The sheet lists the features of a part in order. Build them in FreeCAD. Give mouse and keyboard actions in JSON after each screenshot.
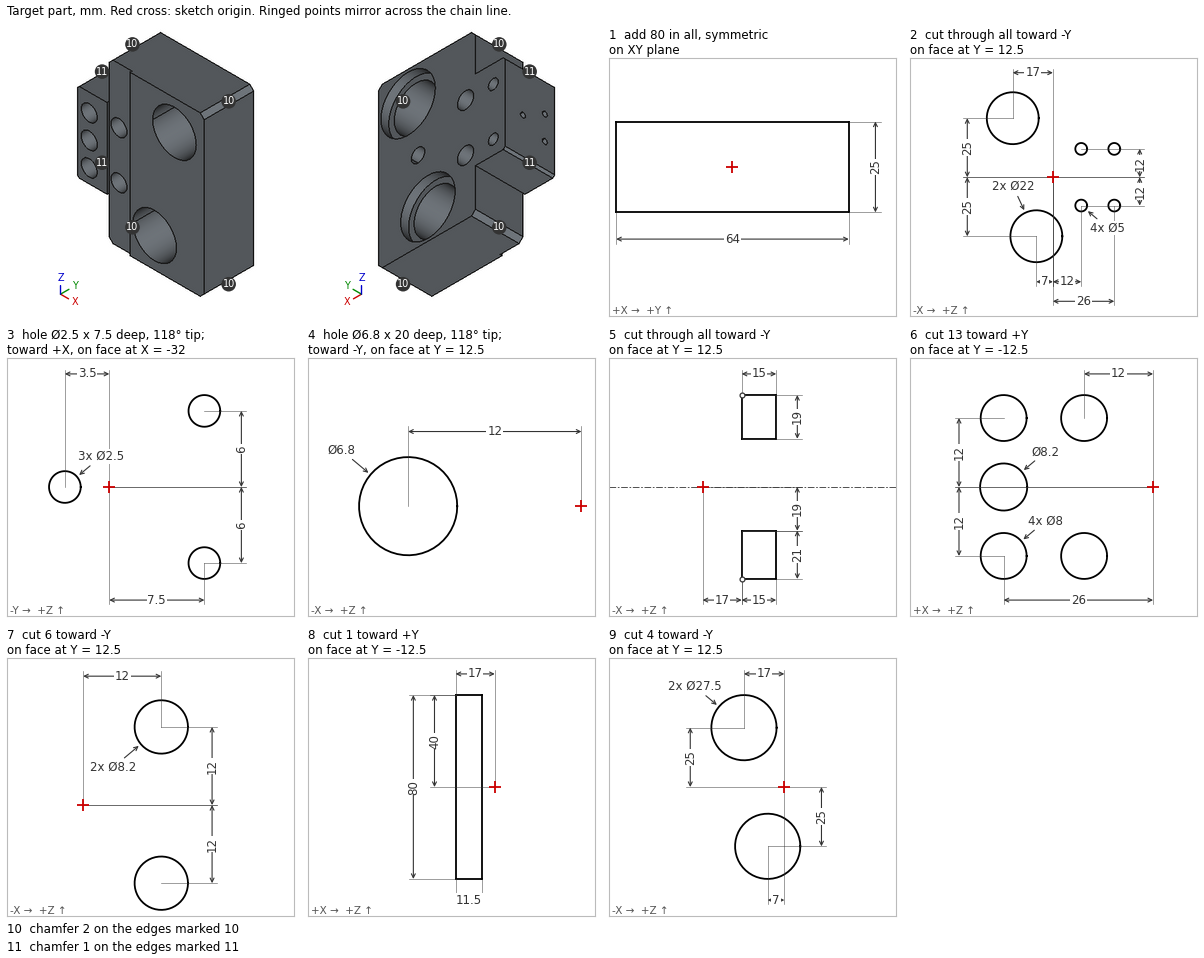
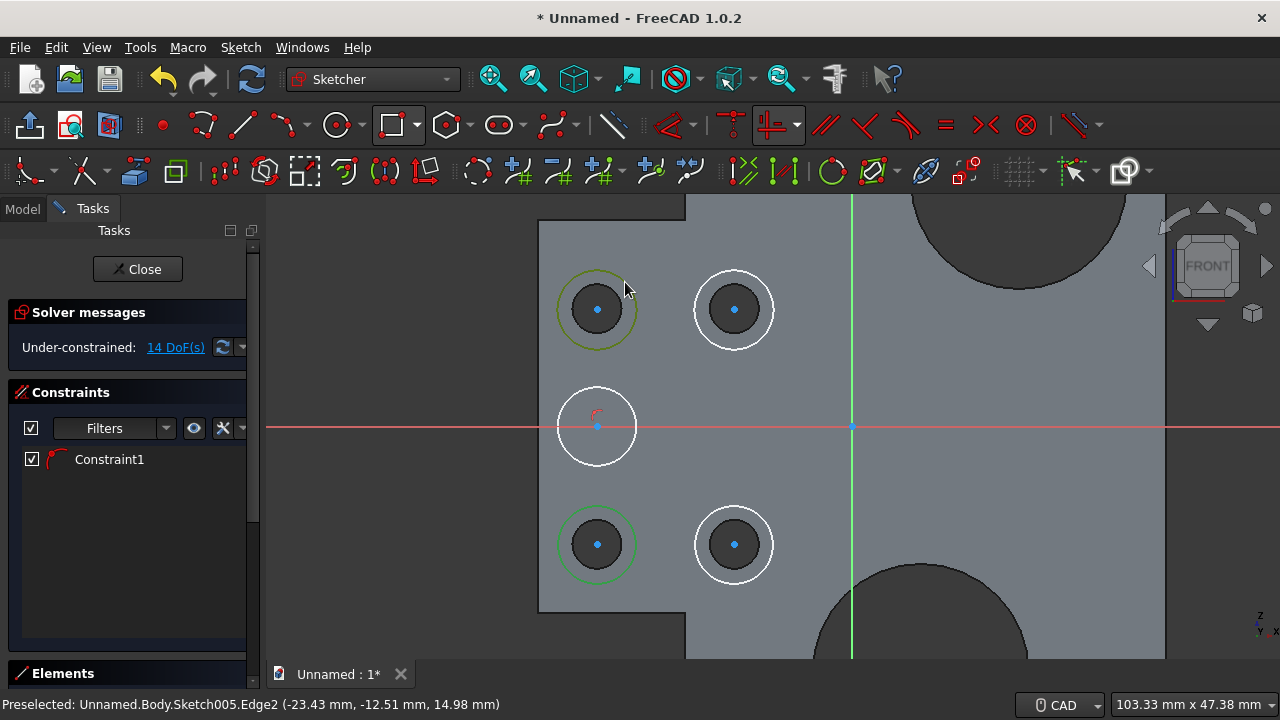
{"action": "left_click", "coordinate": [762, 282]}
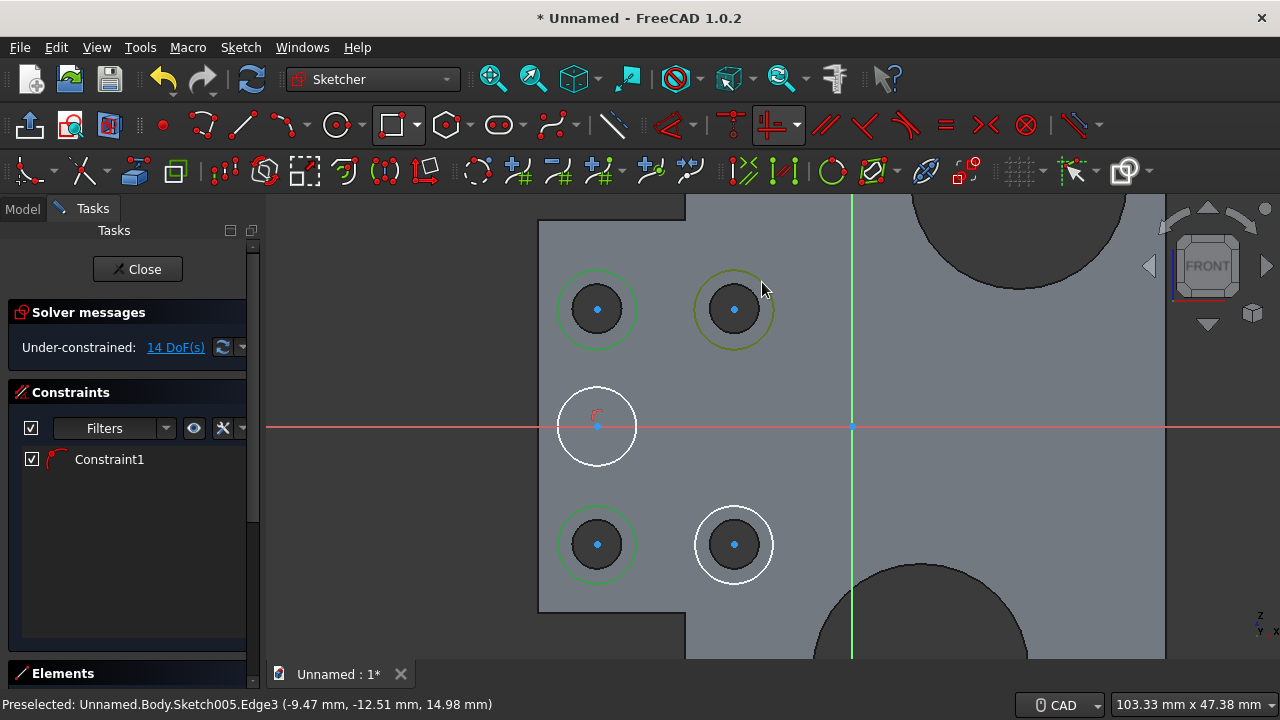
{"action": "left_click", "coordinate": [761, 517]}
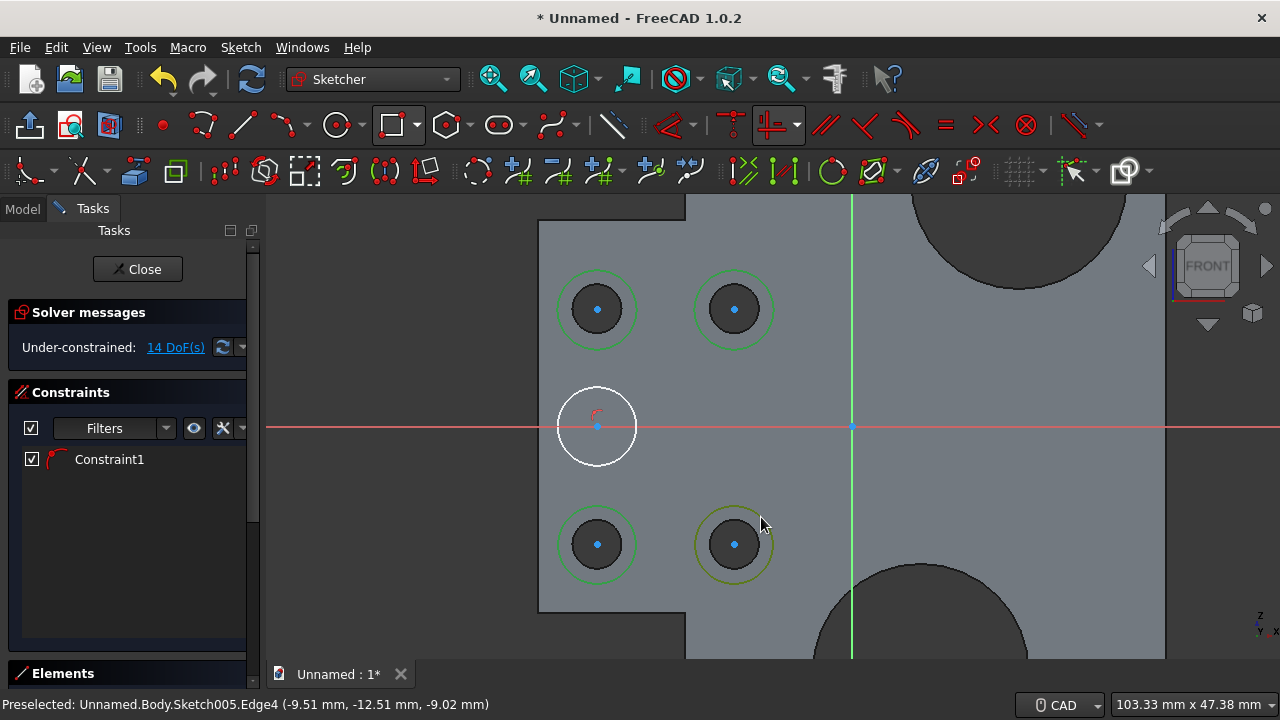
{"action": "left_click", "coordinate": [946, 126]}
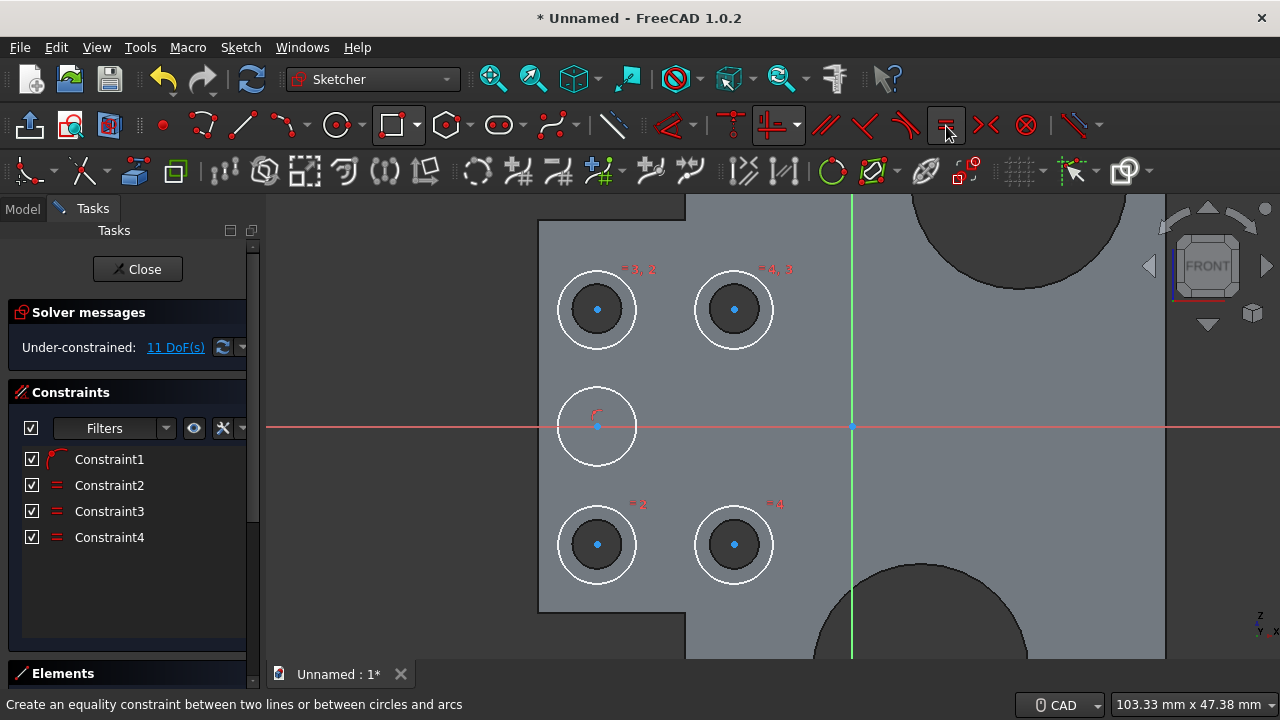
{"action": "left_click", "coordinate": [597, 545]}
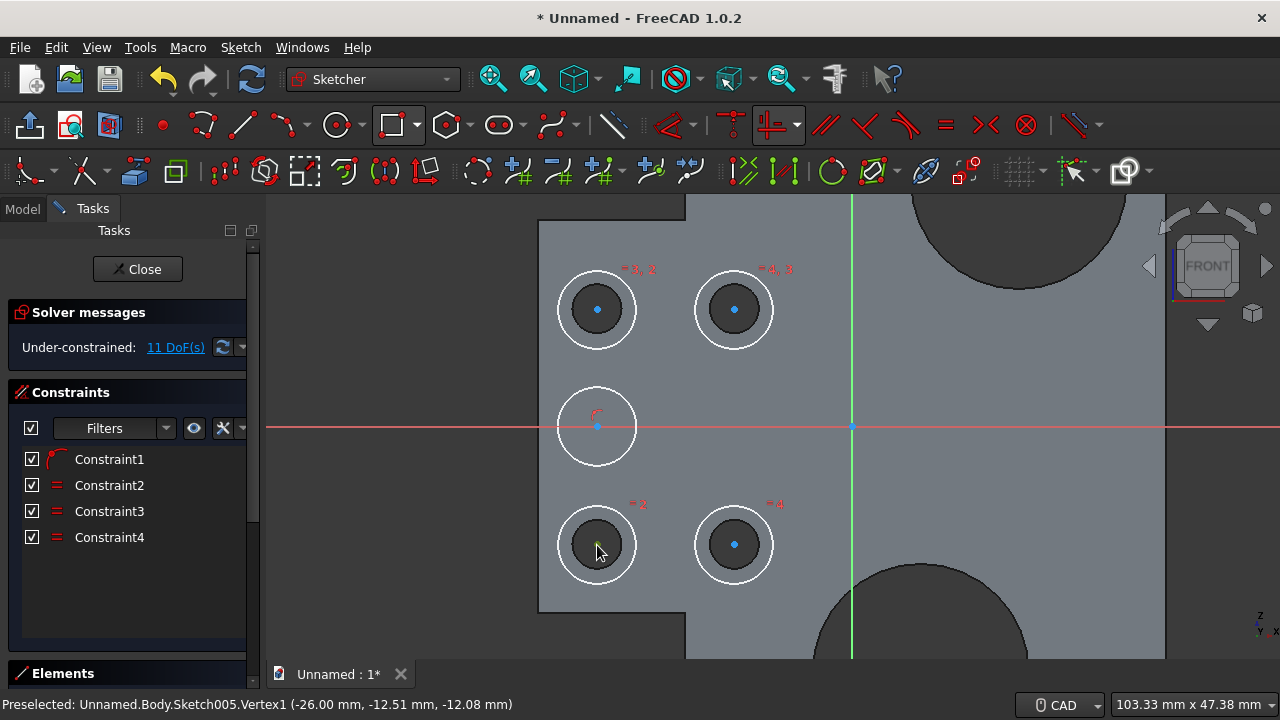
{"action": "left_click", "coordinate": [597, 310]}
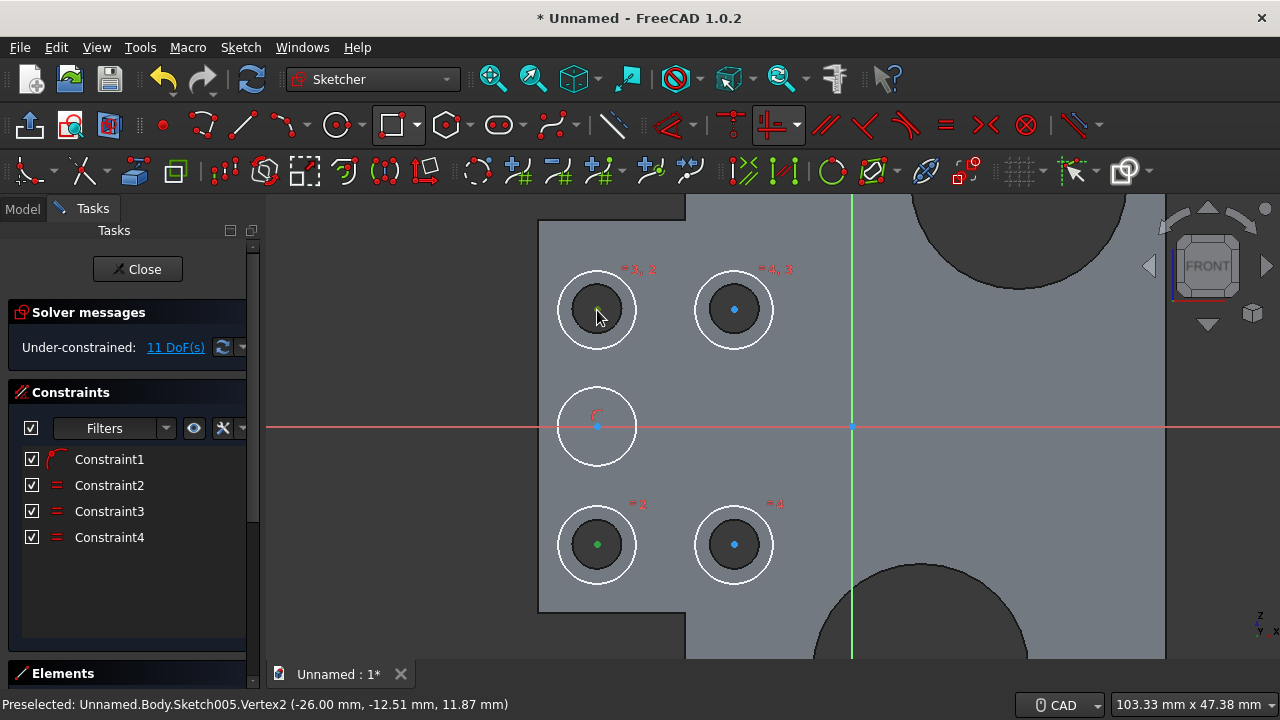
{"action": "left_click", "coordinate": [800, 126]}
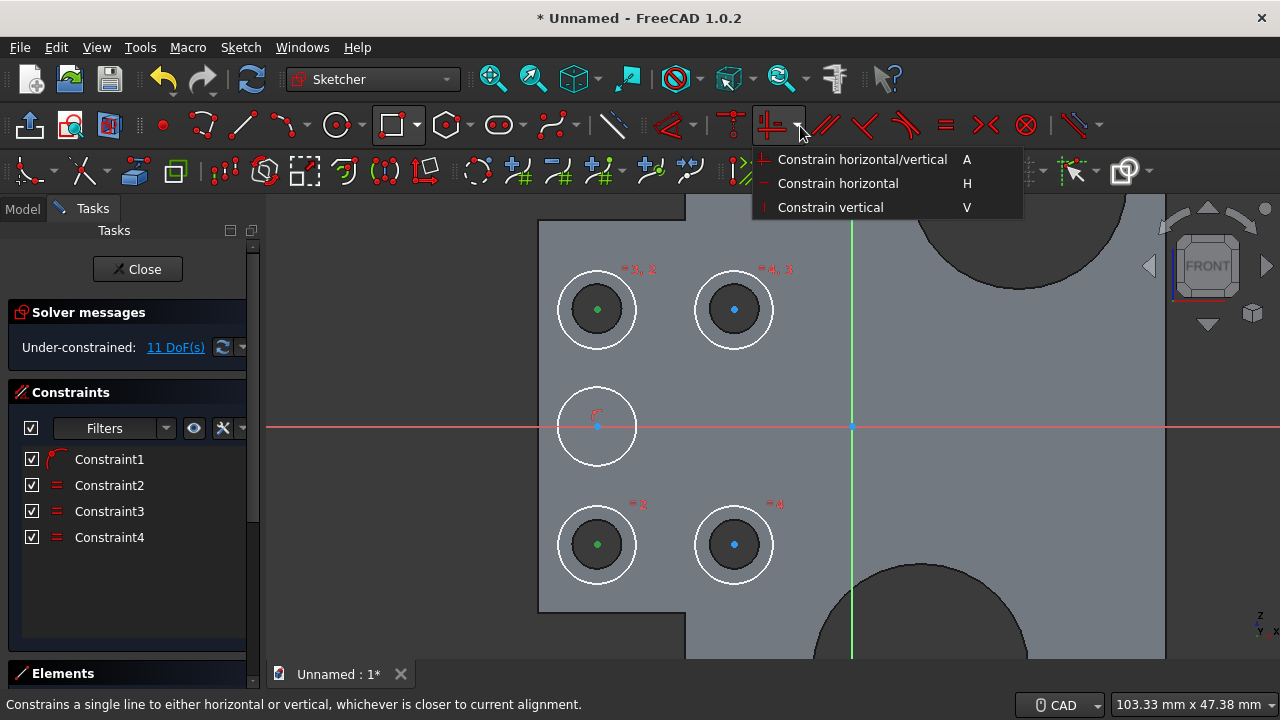
{"action": "left_click", "coordinate": [888, 207]}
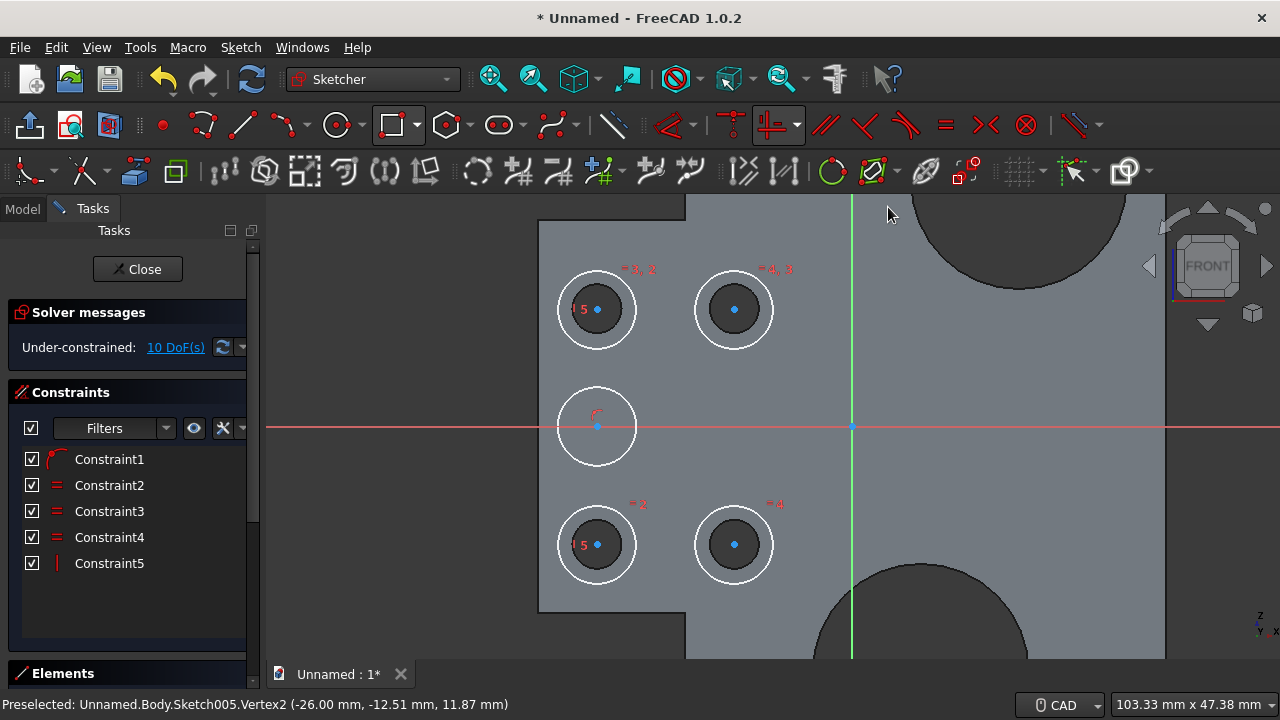
{"action": "left_click", "coordinate": [597, 310]}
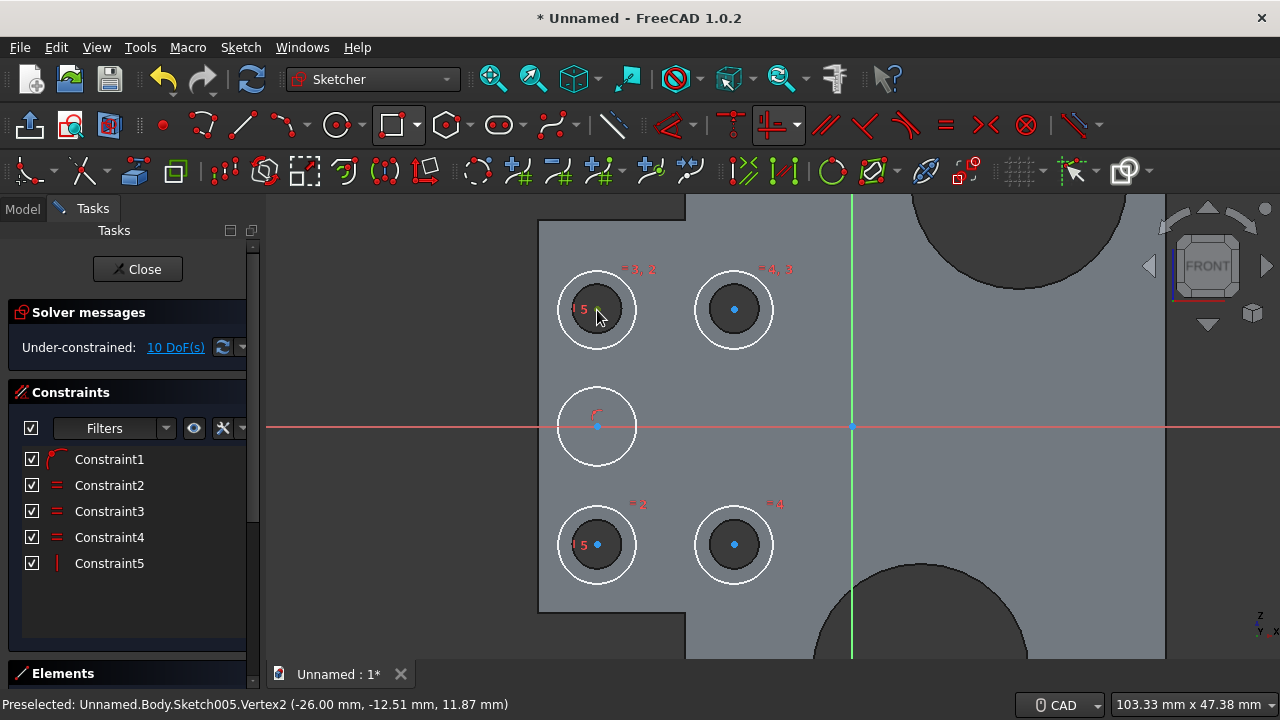
{"action": "left_click", "coordinate": [734, 310]}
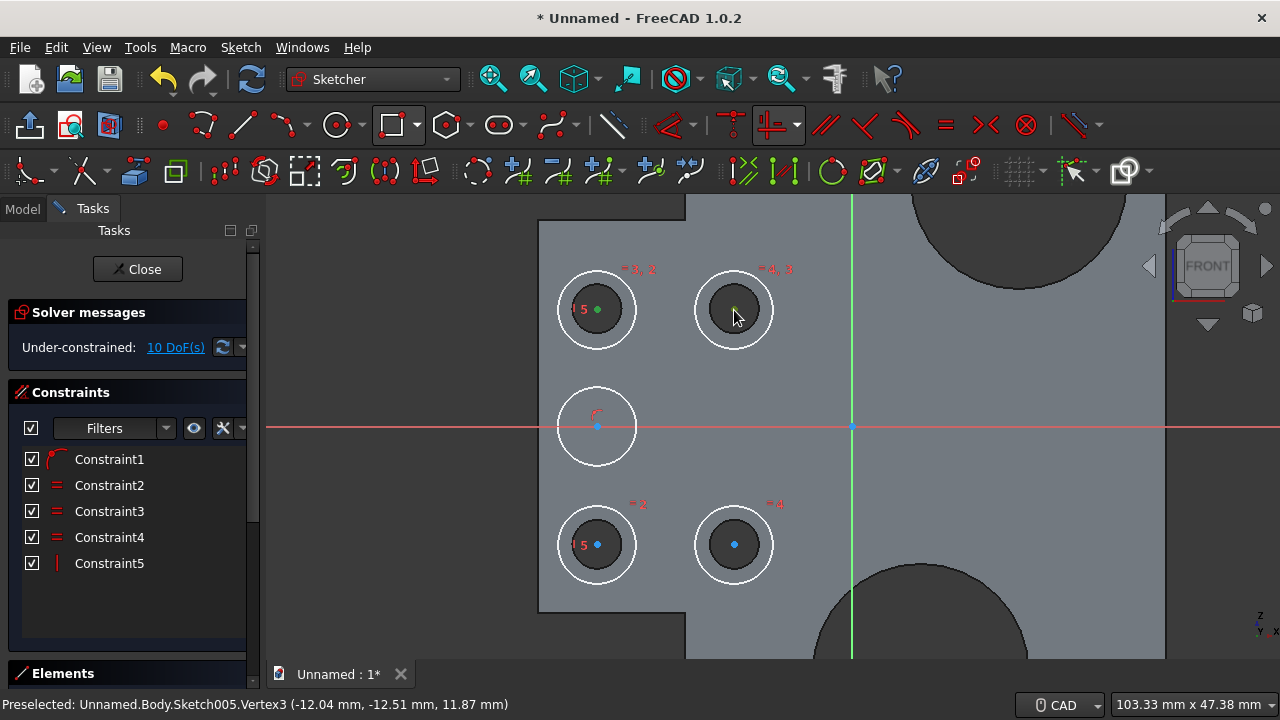
{"action": "left_click", "coordinate": [800, 126]}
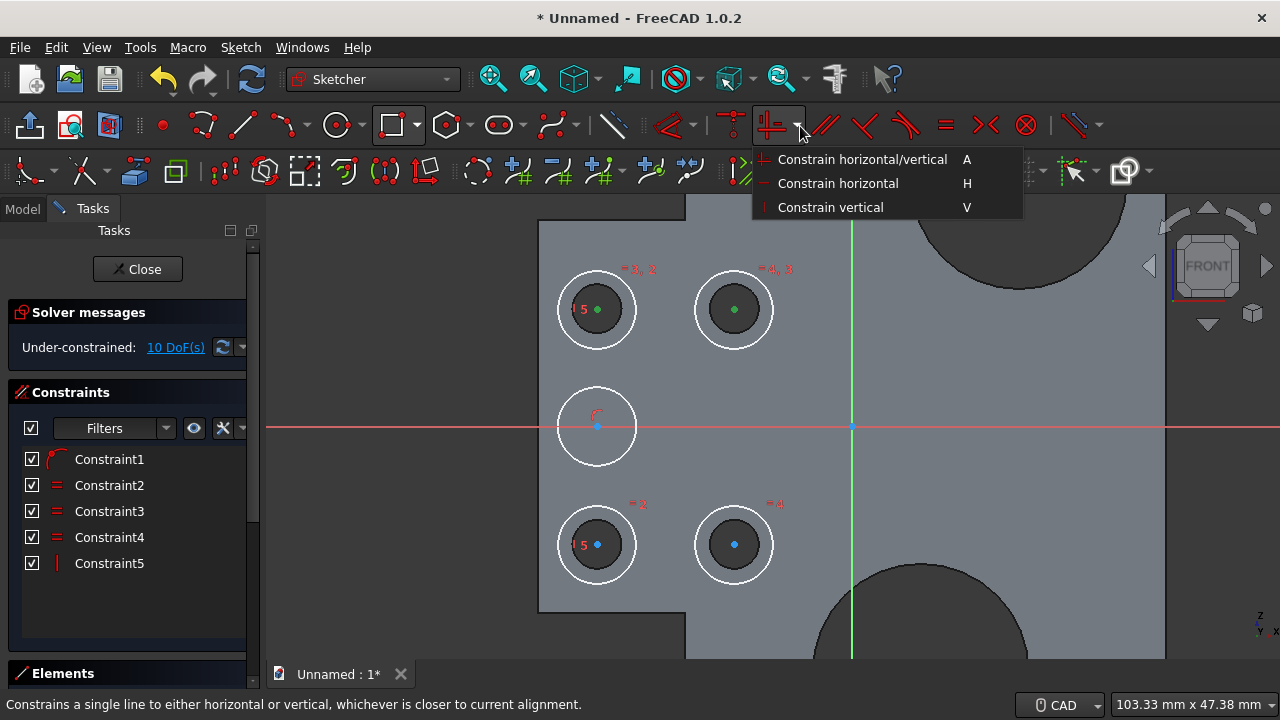
{"action": "left_click", "coordinate": [888, 183]}